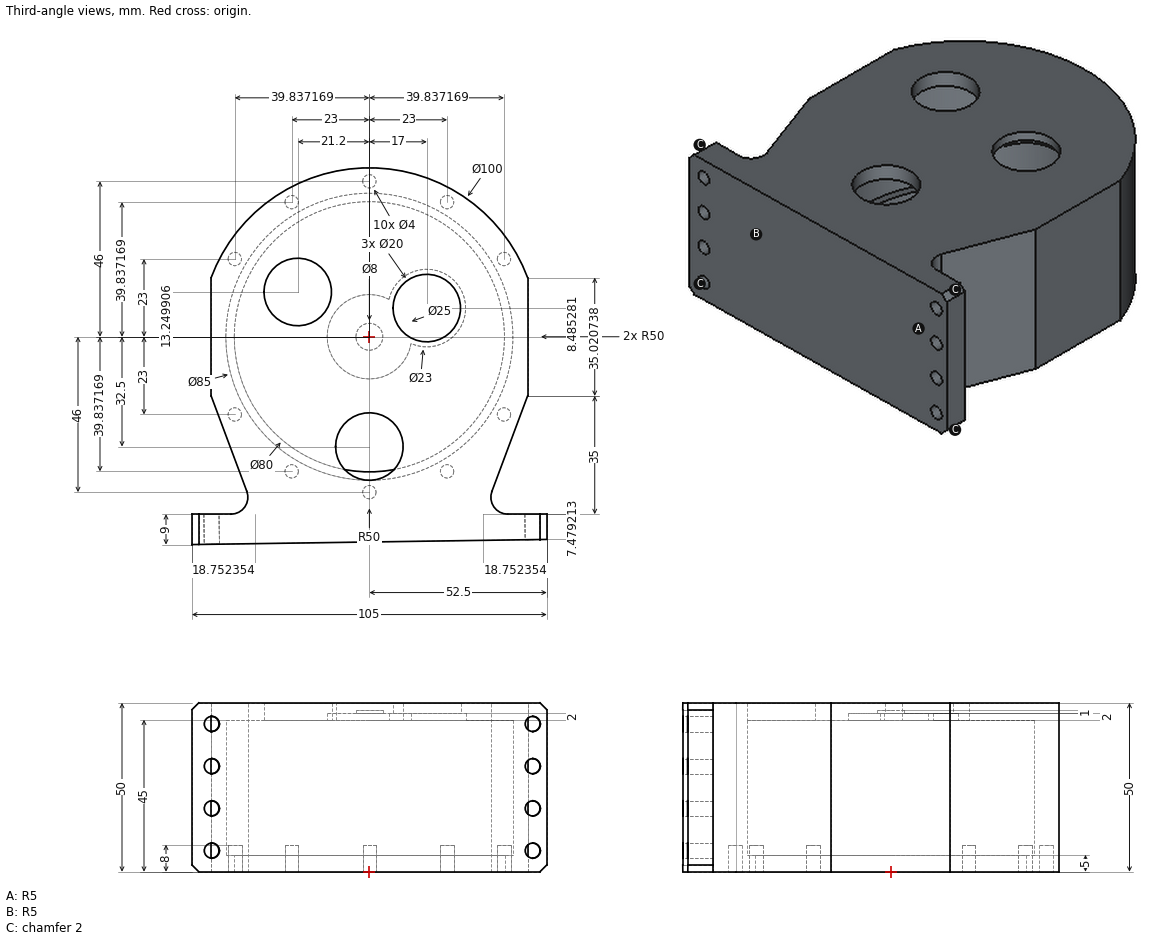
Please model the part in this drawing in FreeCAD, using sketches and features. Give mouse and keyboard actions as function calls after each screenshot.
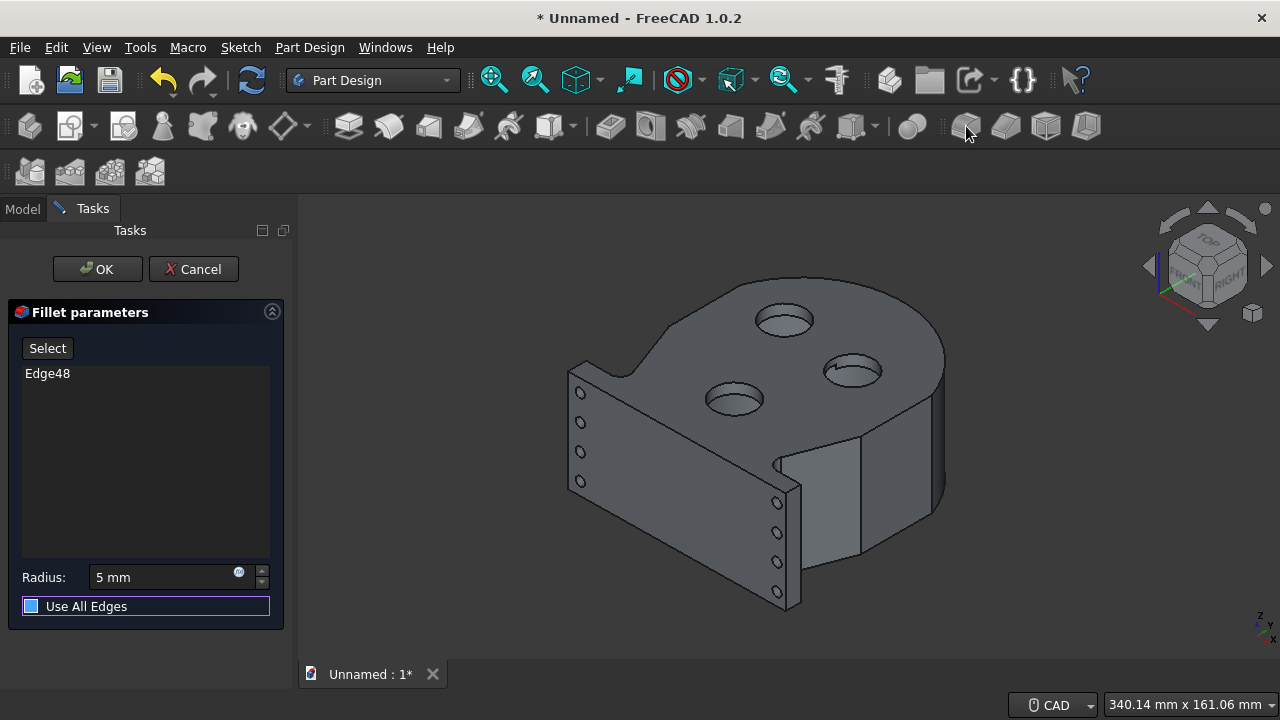
click(98, 269)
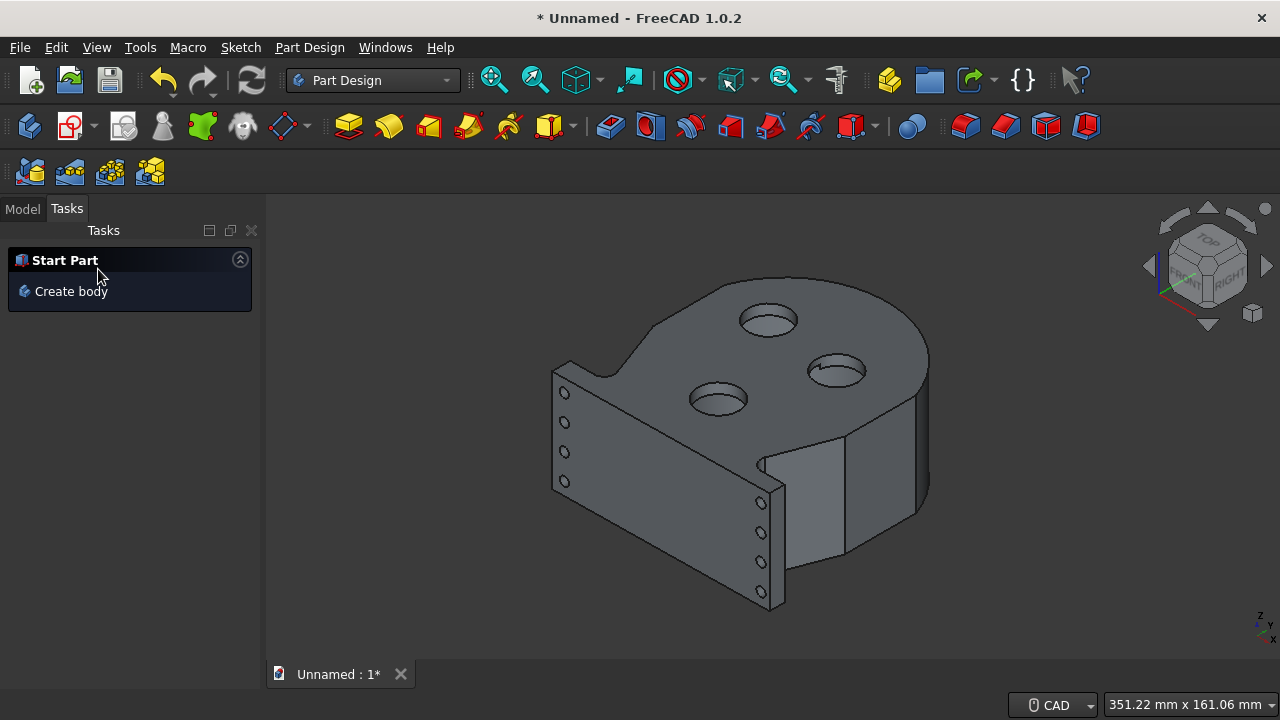
click(777, 488)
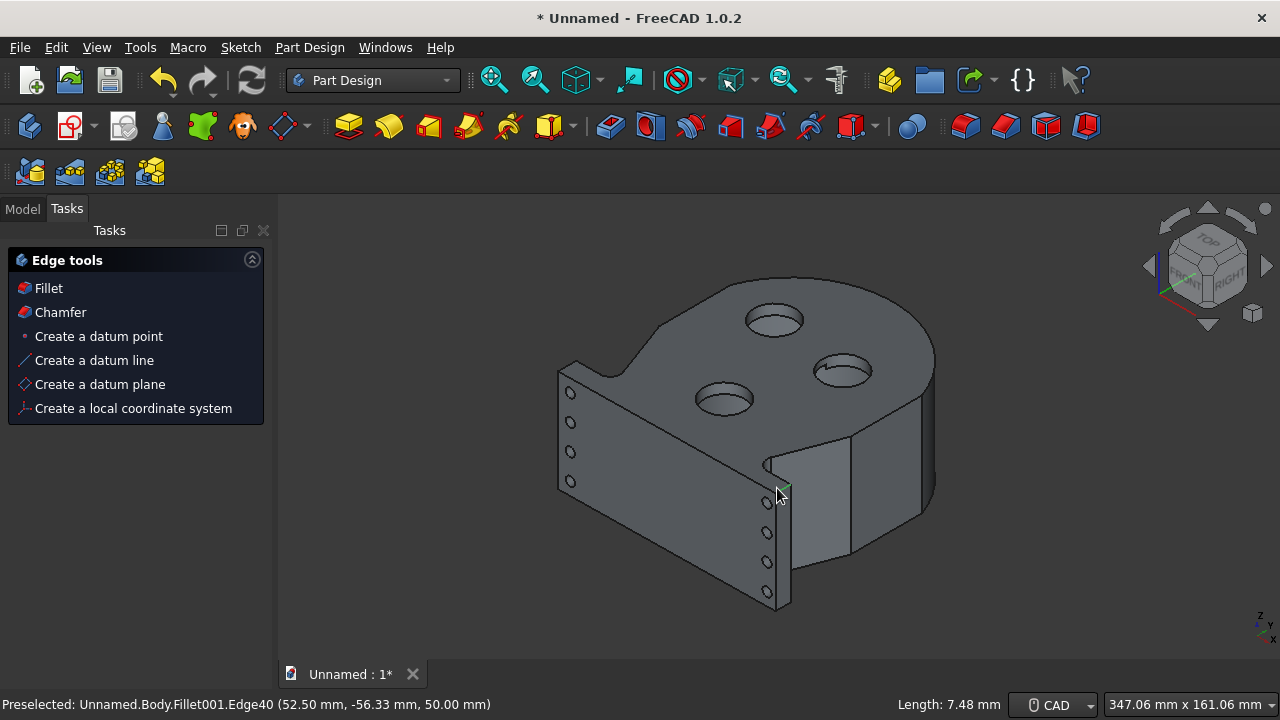
key(2)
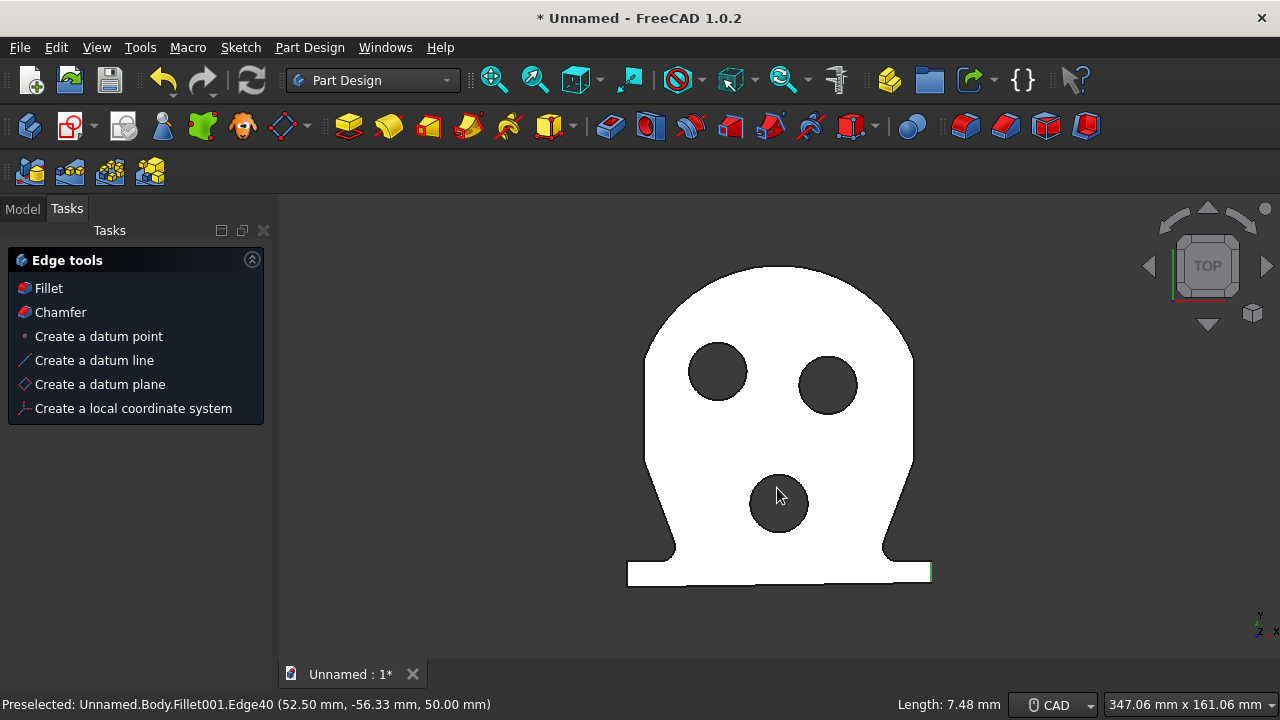
click(627, 573, ctrl)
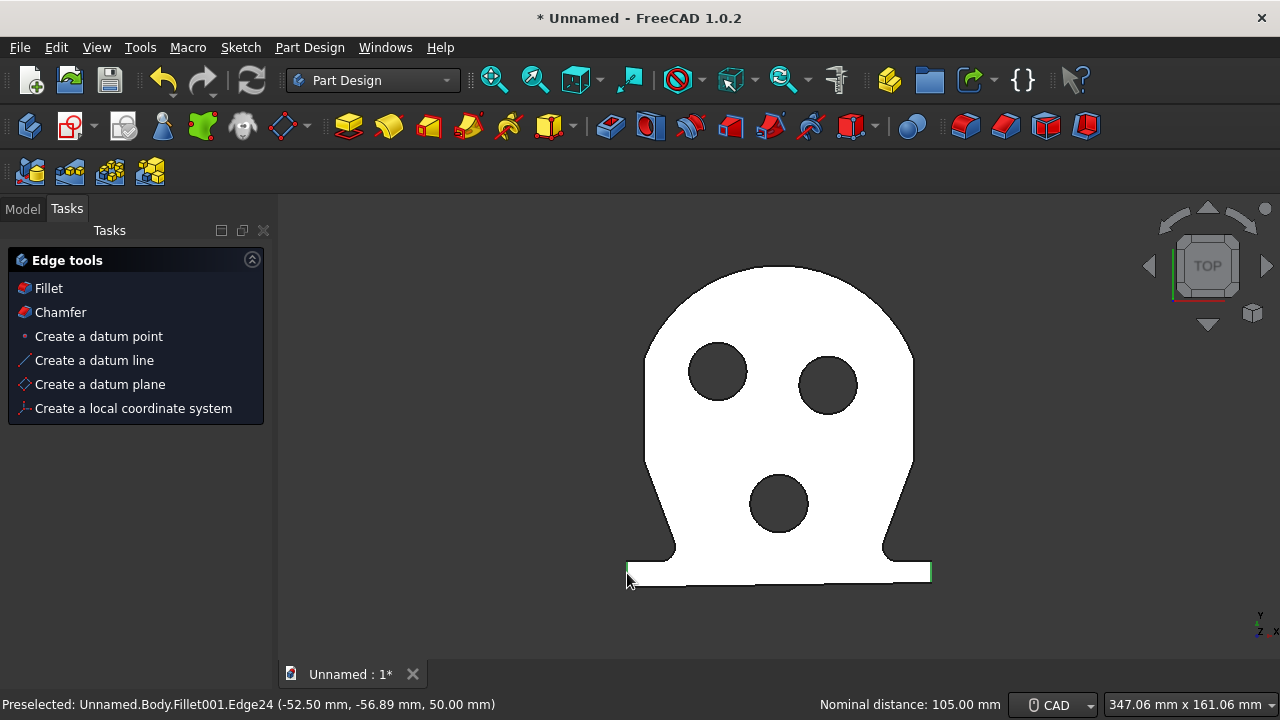
scroll(931, 571, up, 4)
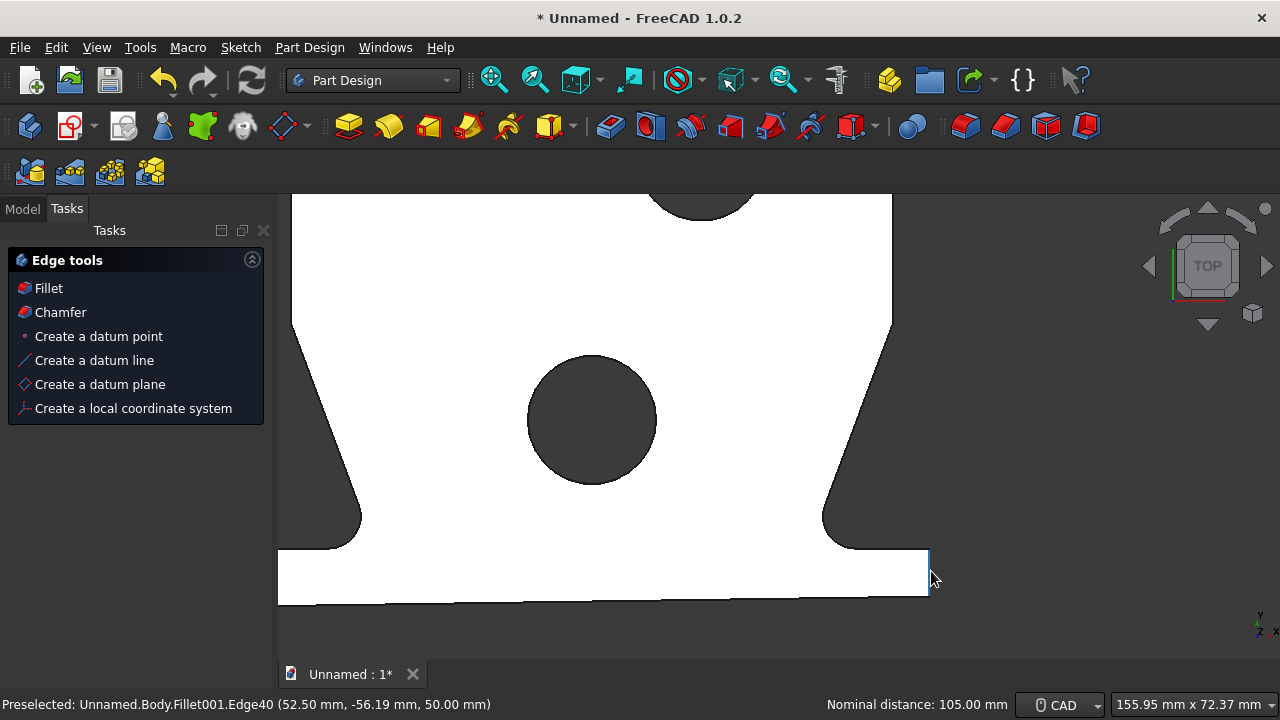
click(496, 80)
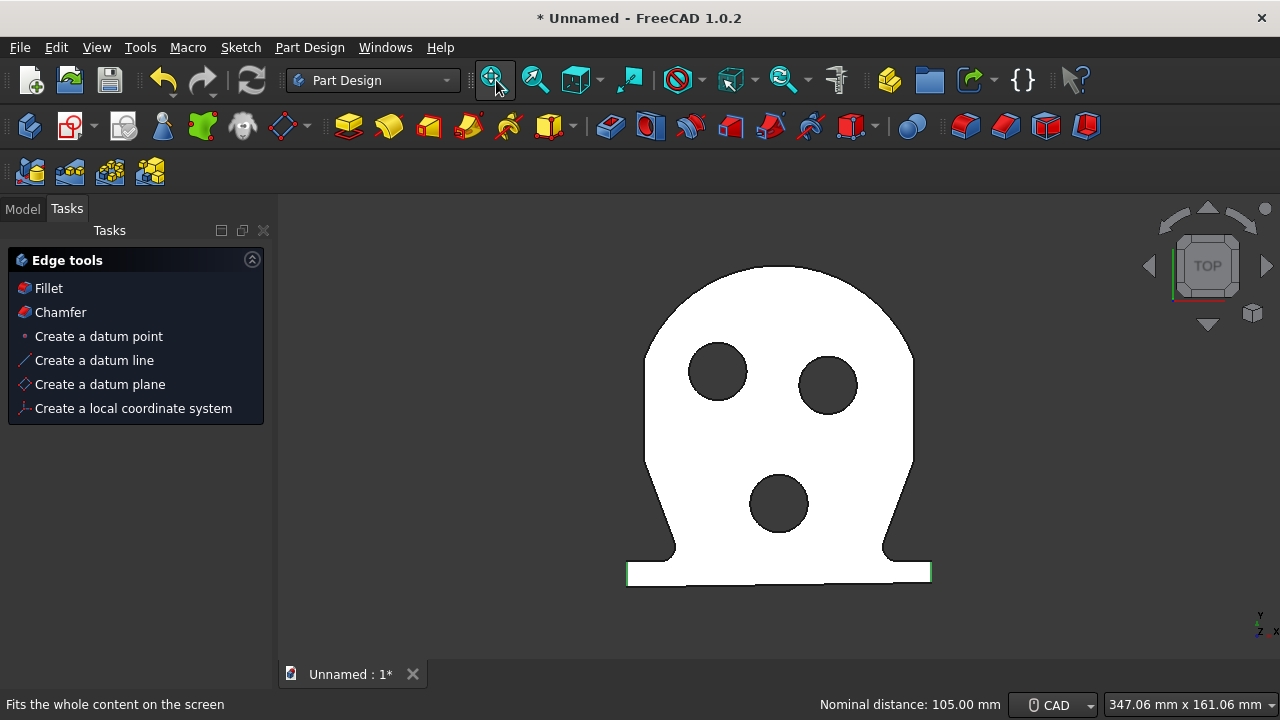
key(0)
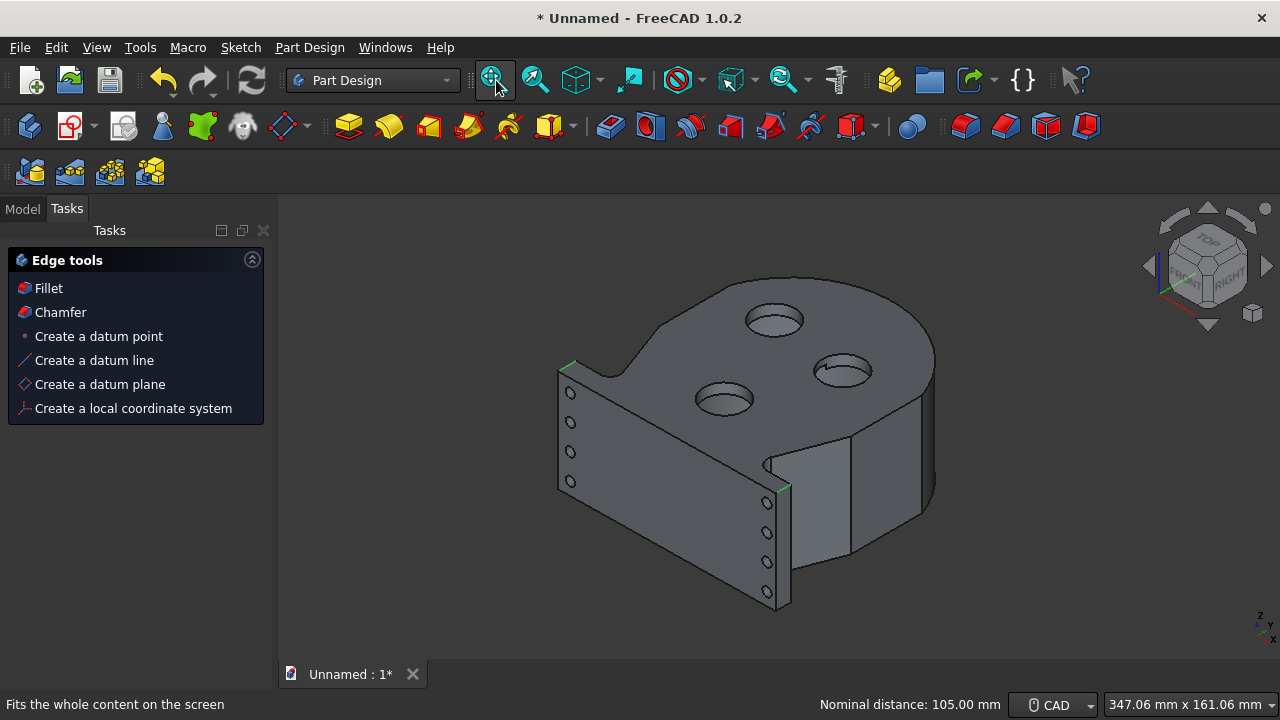
scroll(783, 606, up, 4)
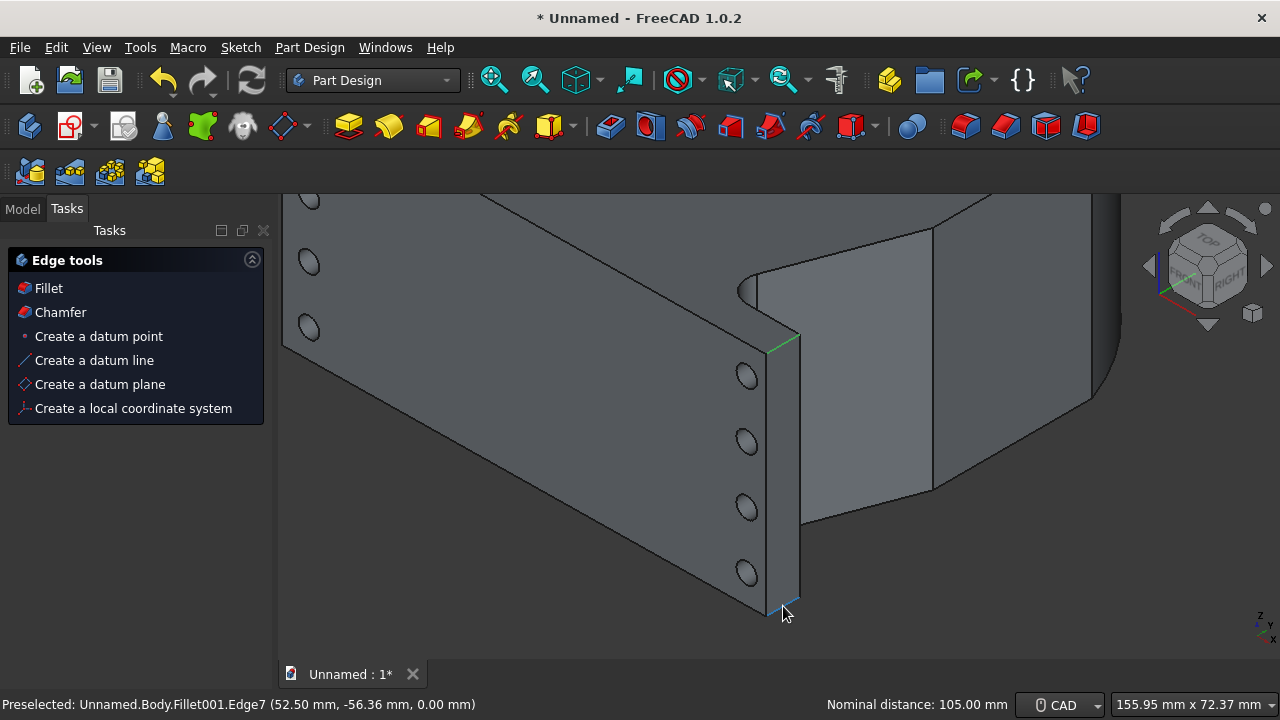
click(496, 80)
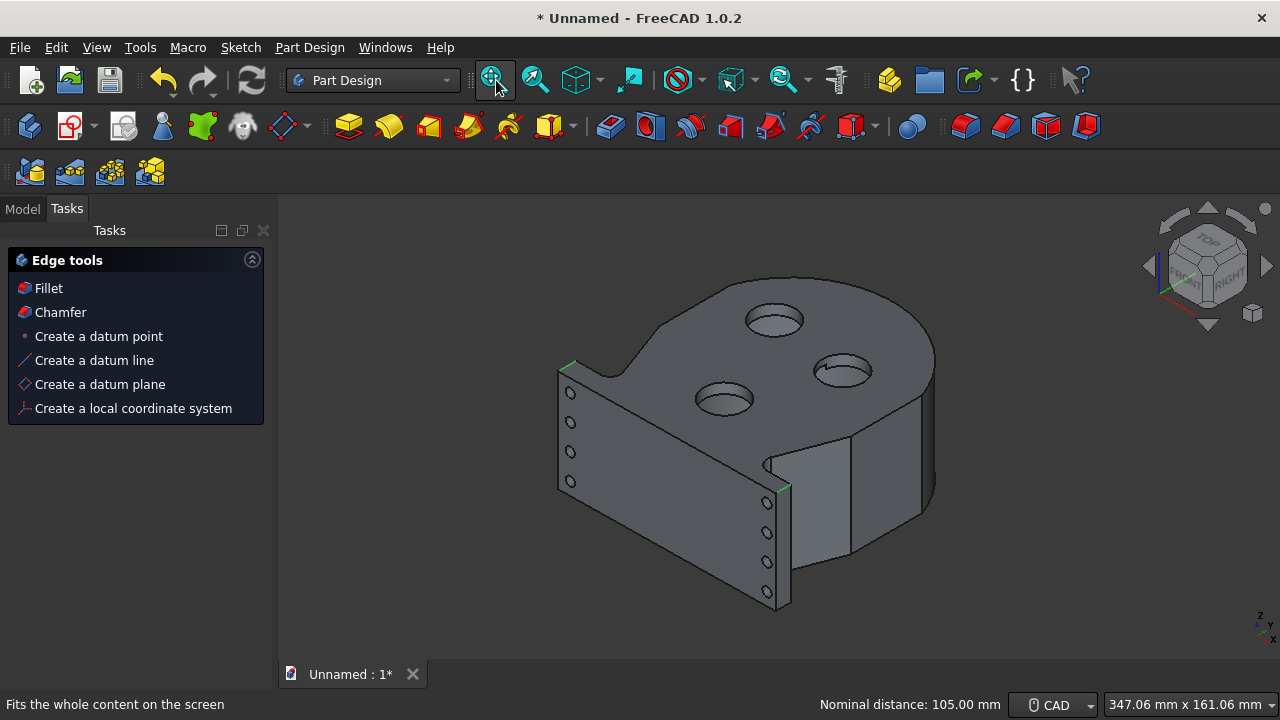
key(1)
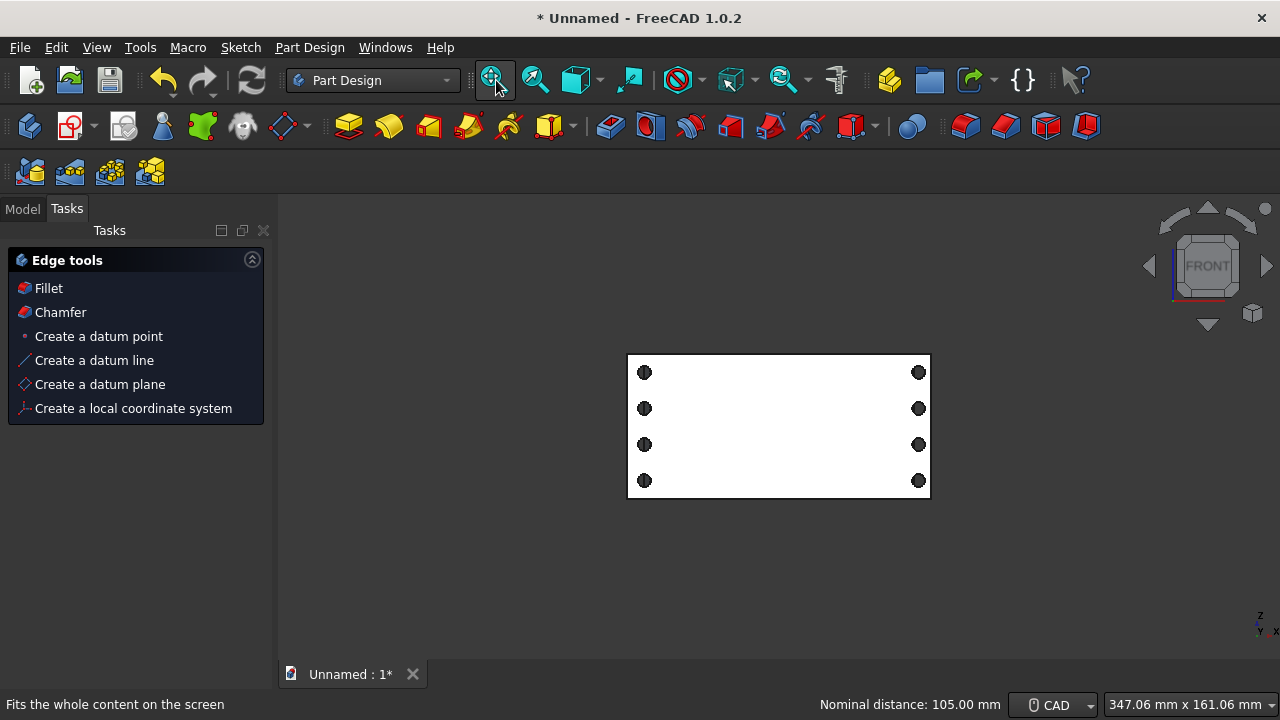
click(496, 80)